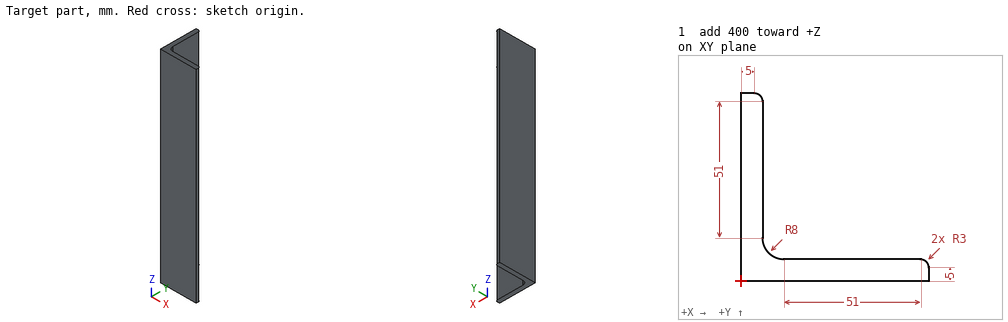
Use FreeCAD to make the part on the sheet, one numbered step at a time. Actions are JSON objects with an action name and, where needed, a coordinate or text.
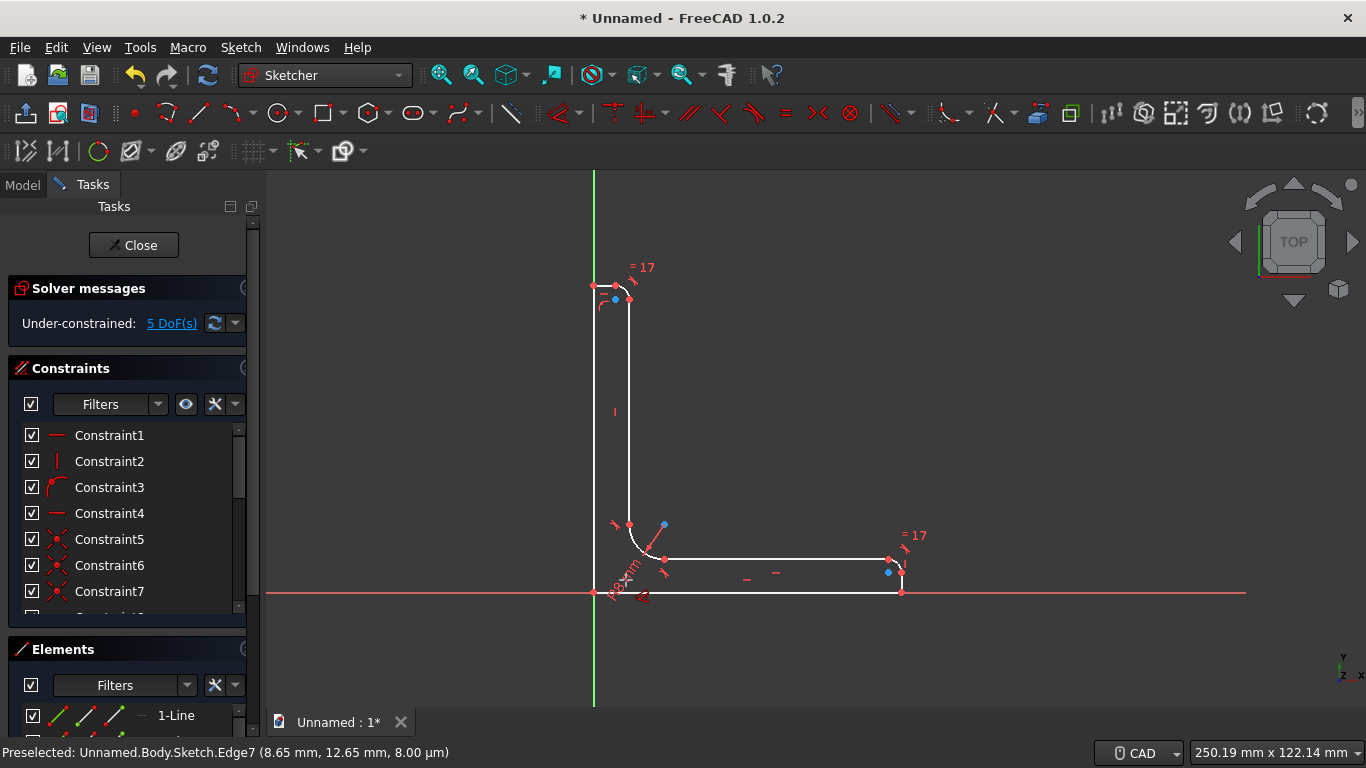
{"action": "scroll", "coordinate": [625, 290], "scroll_direction": "up", "scroll_amount": 6}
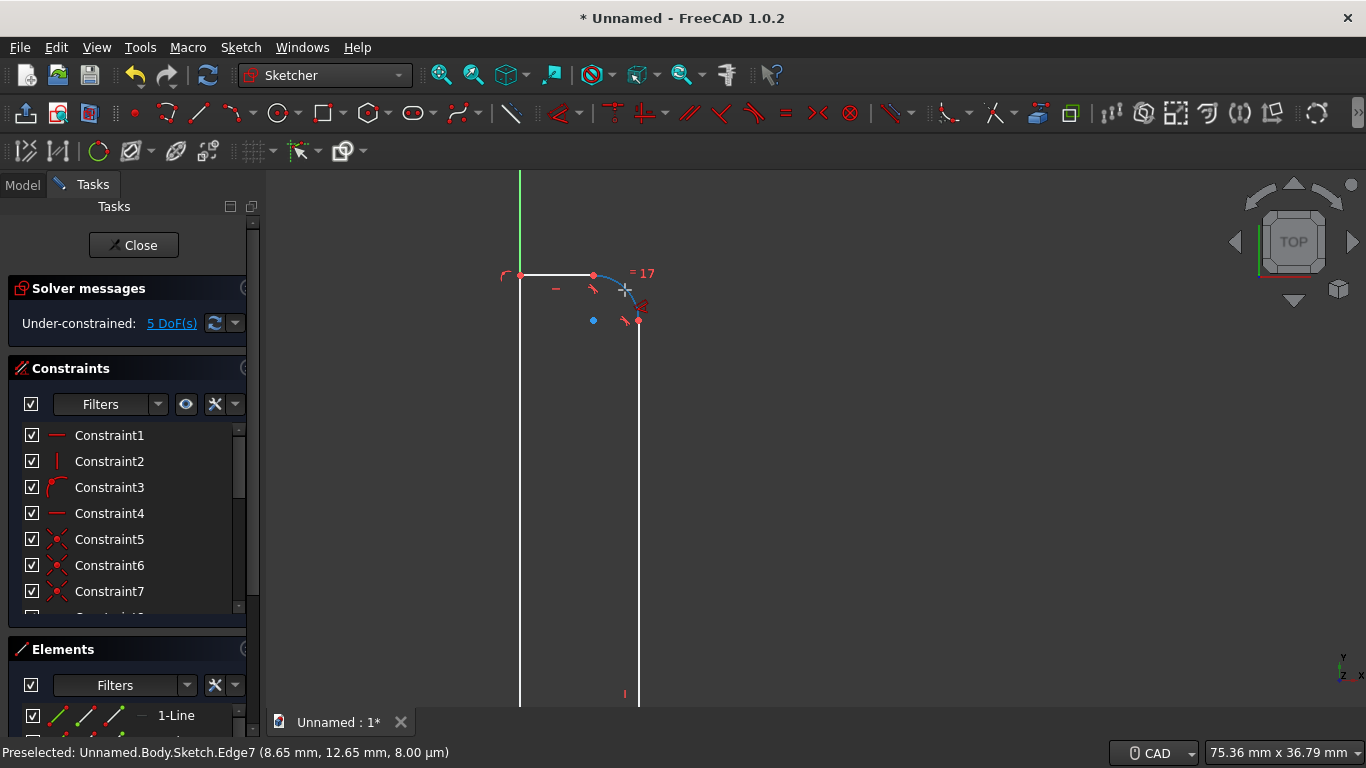
{"action": "left_click", "coordinate": [625, 289]}
{"action": "left_click", "coordinate": [648, 266]}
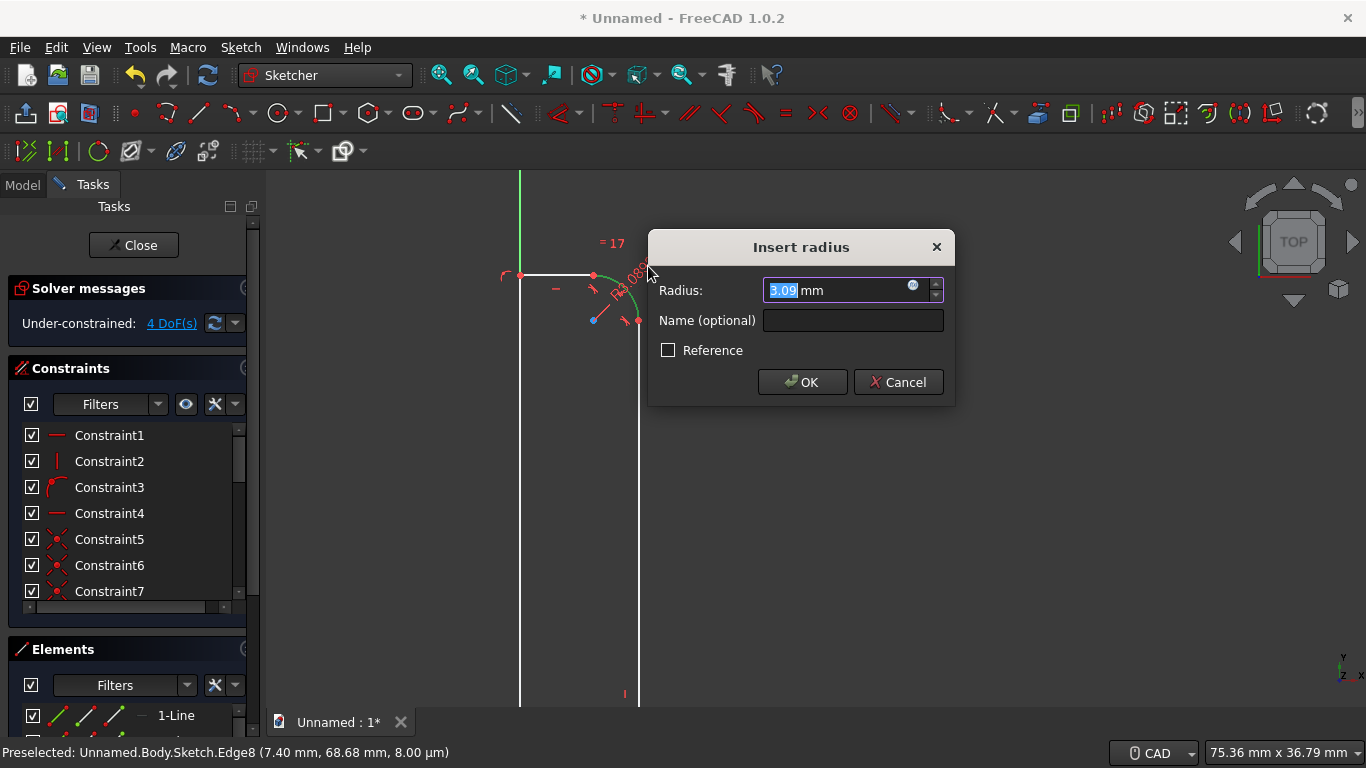
{"action": "type", "text": "3"}
{"action": "key", "text": "Return"}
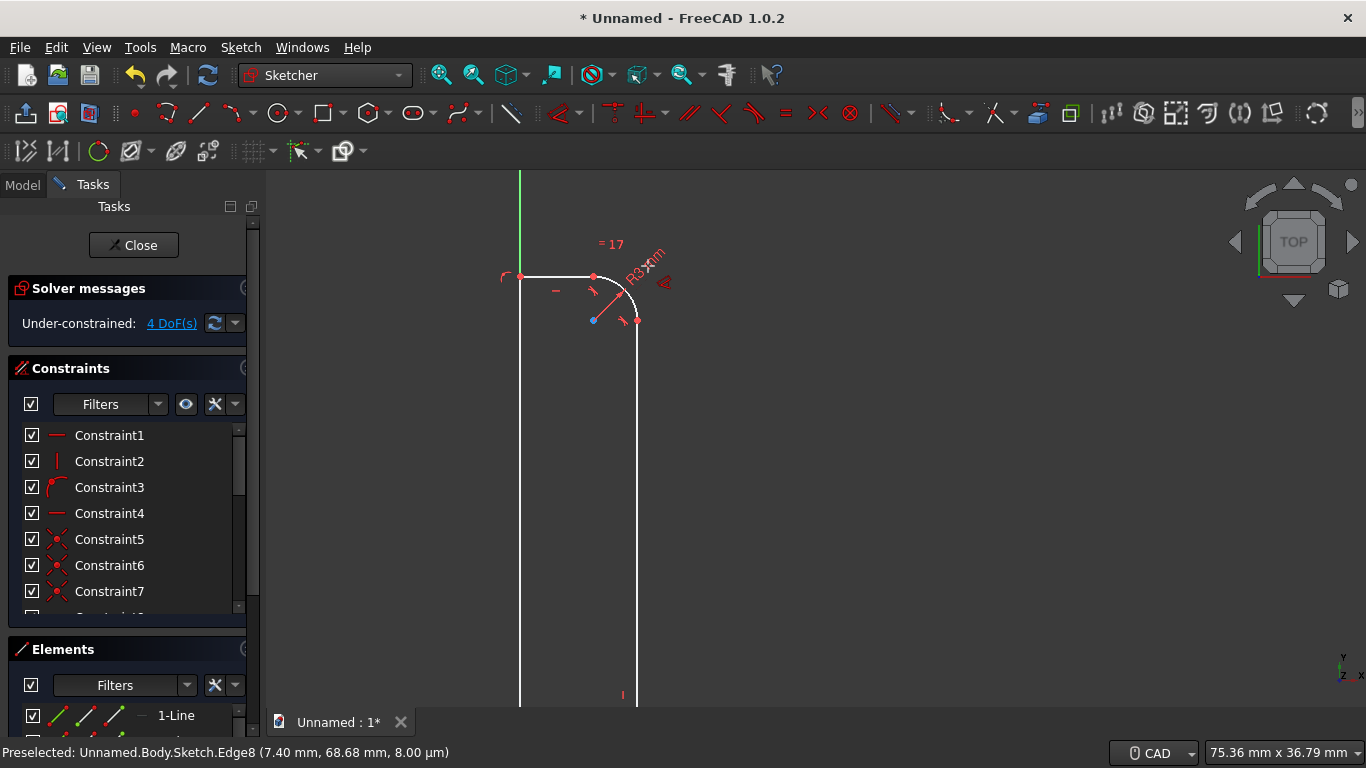
{"action": "left_click", "coordinate": [572, 277]}
{"action": "left_click", "coordinate": [557, 243]}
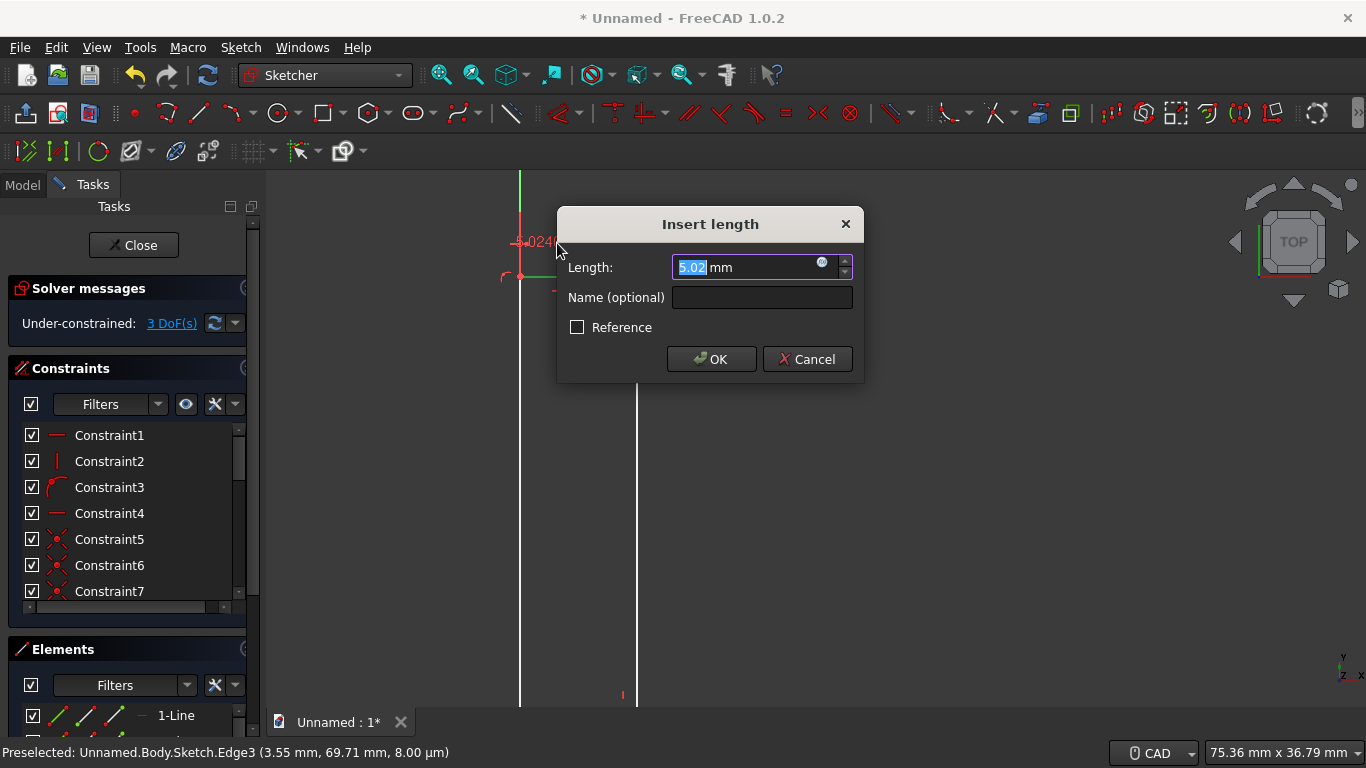
{"action": "type", "text": "5"}
{"action": "key", "text": "Return"}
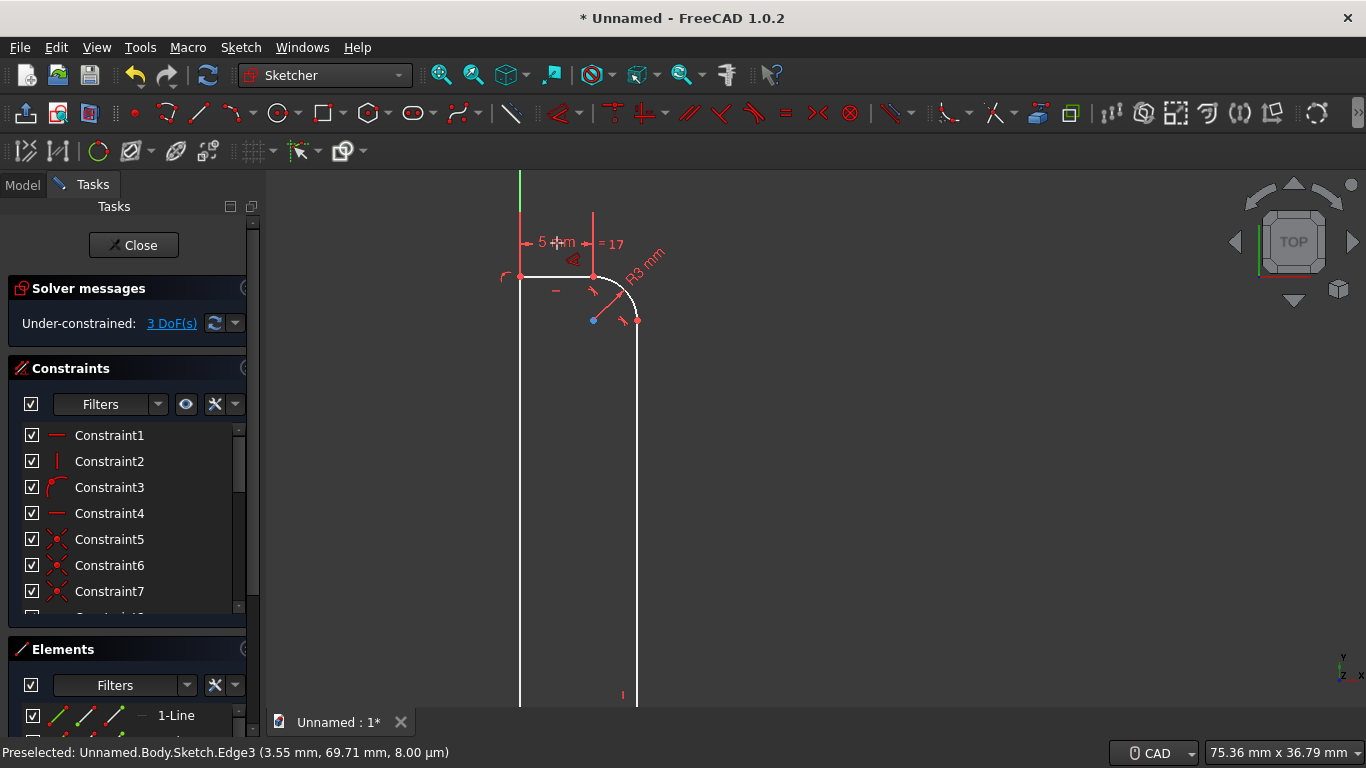
{"action": "scroll", "coordinate": [625, 290], "scroll_direction": "down", "scroll_amount": 6}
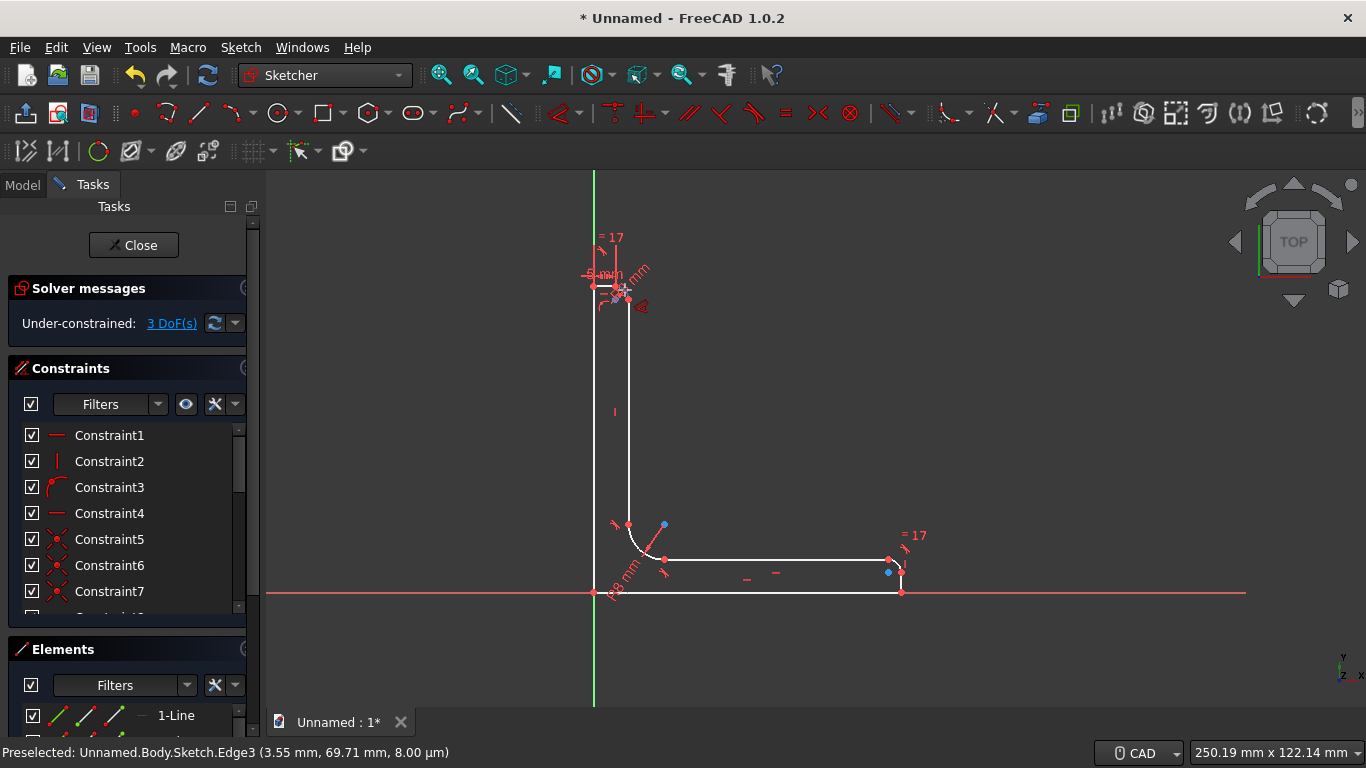
{"action": "scroll", "coordinate": [901, 587], "scroll_direction": "up", "scroll_amount": 5}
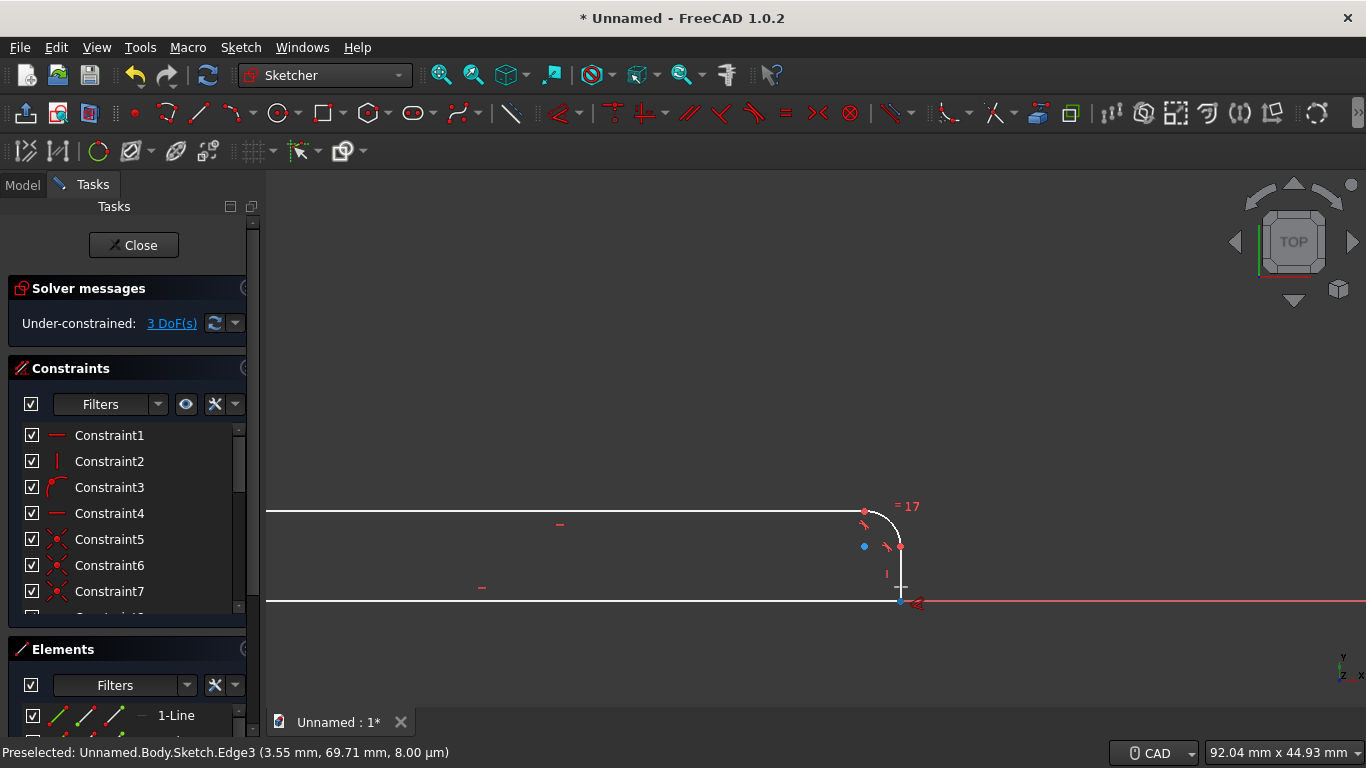
{"action": "left_click", "coordinate": [901, 585]}
{"action": "left_click", "coordinate": [935, 574]}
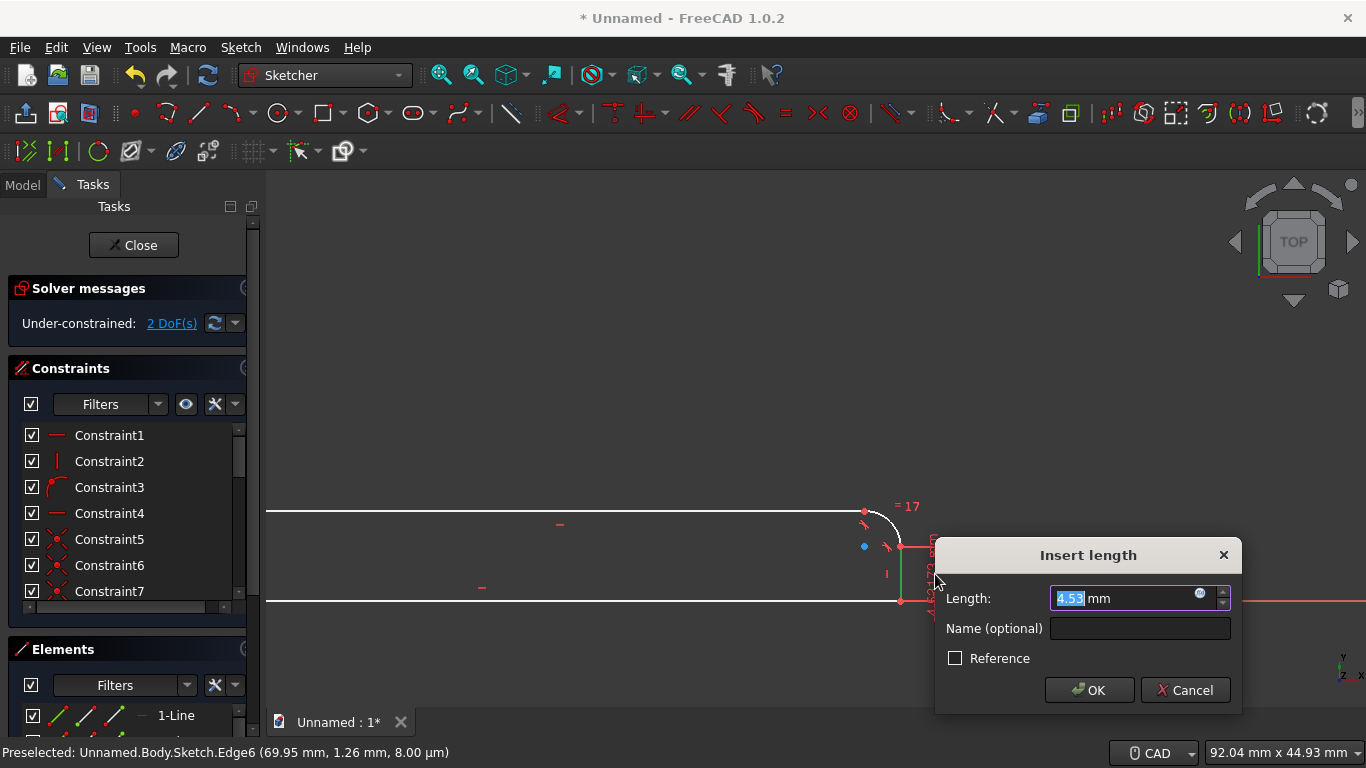
{"action": "type", "text": "5"}
{"action": "key", "text": "Return"}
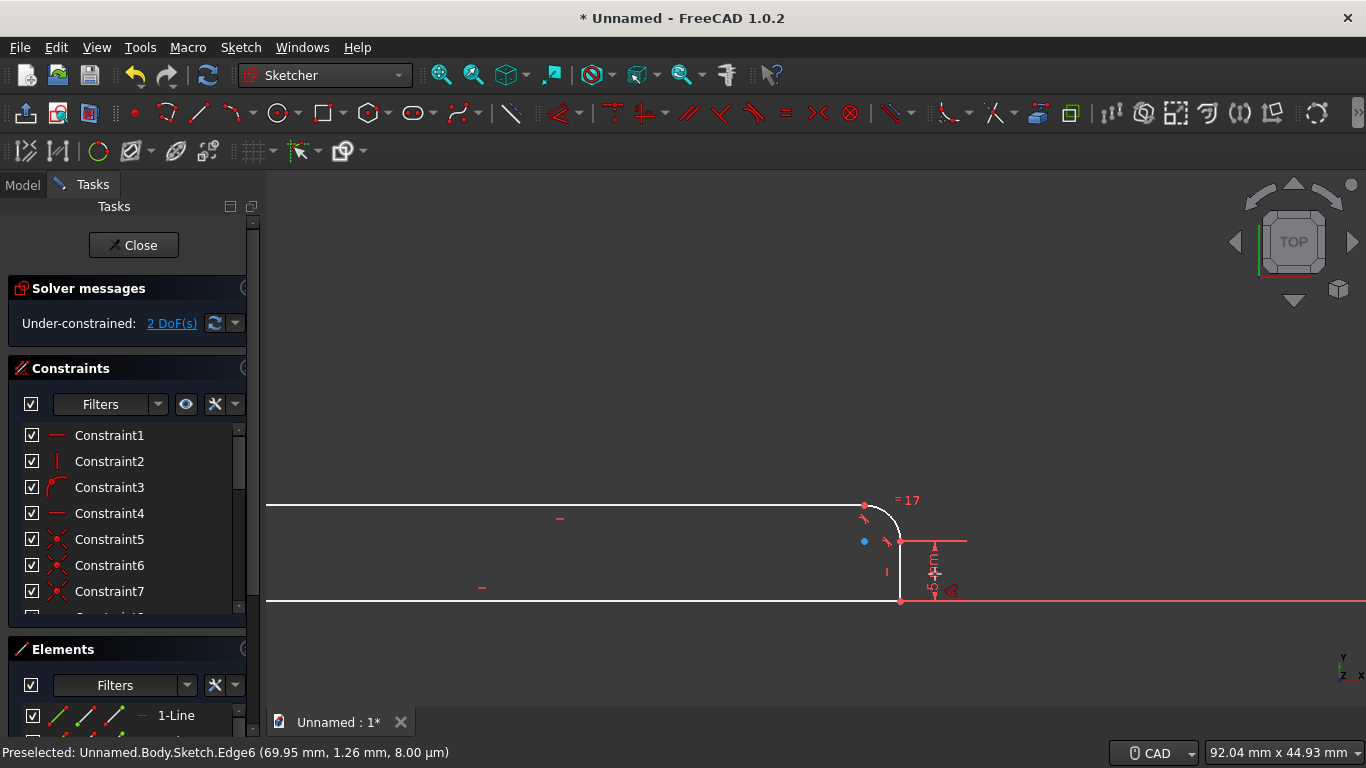
{"action": "left_click", "coordinate": [682, 505]}
{"action": "left_click", "coordinate": [579, 539]}